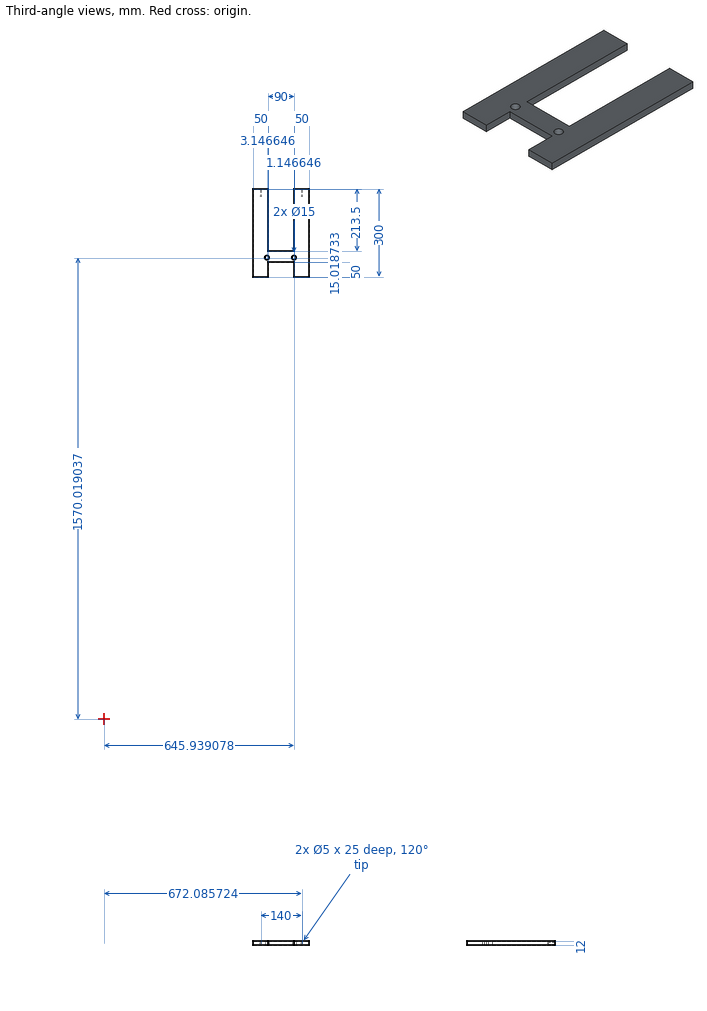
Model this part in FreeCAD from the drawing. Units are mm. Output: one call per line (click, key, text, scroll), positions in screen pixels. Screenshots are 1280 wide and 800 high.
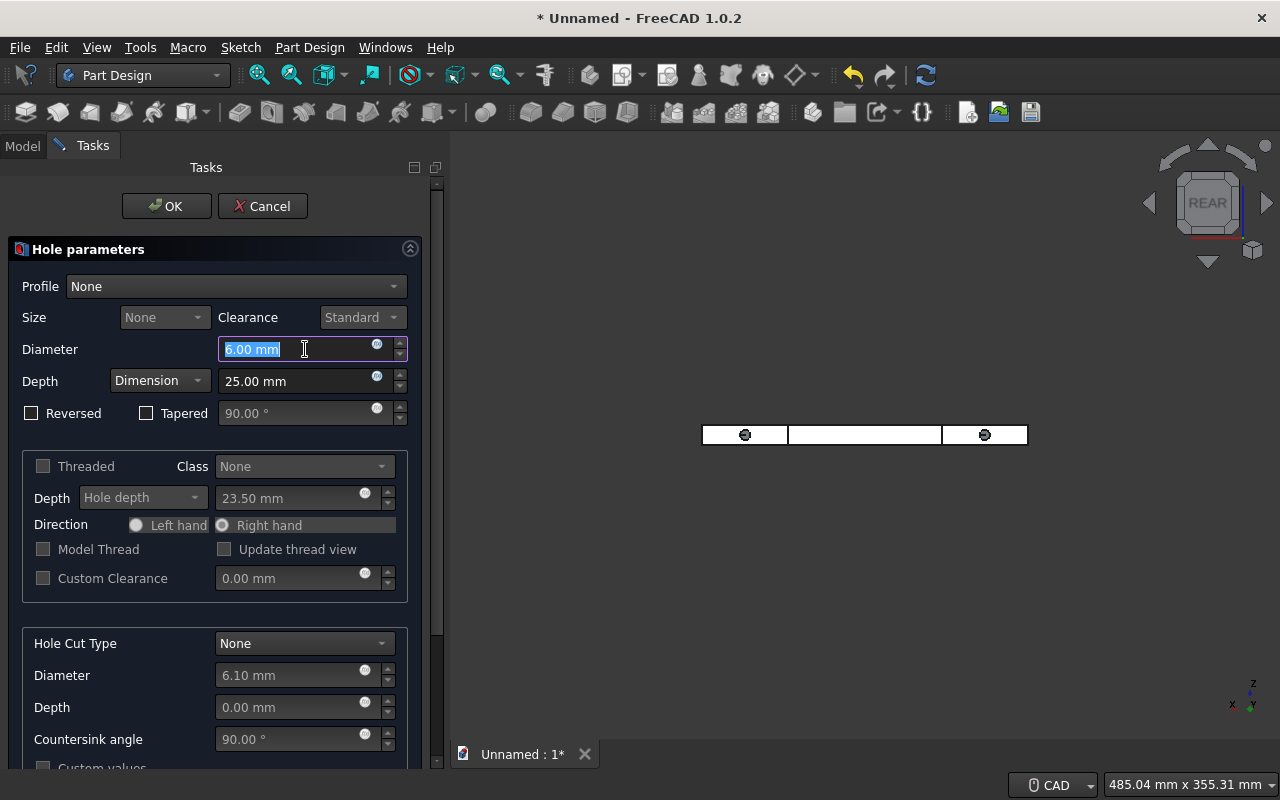
text(5)
key(Tab)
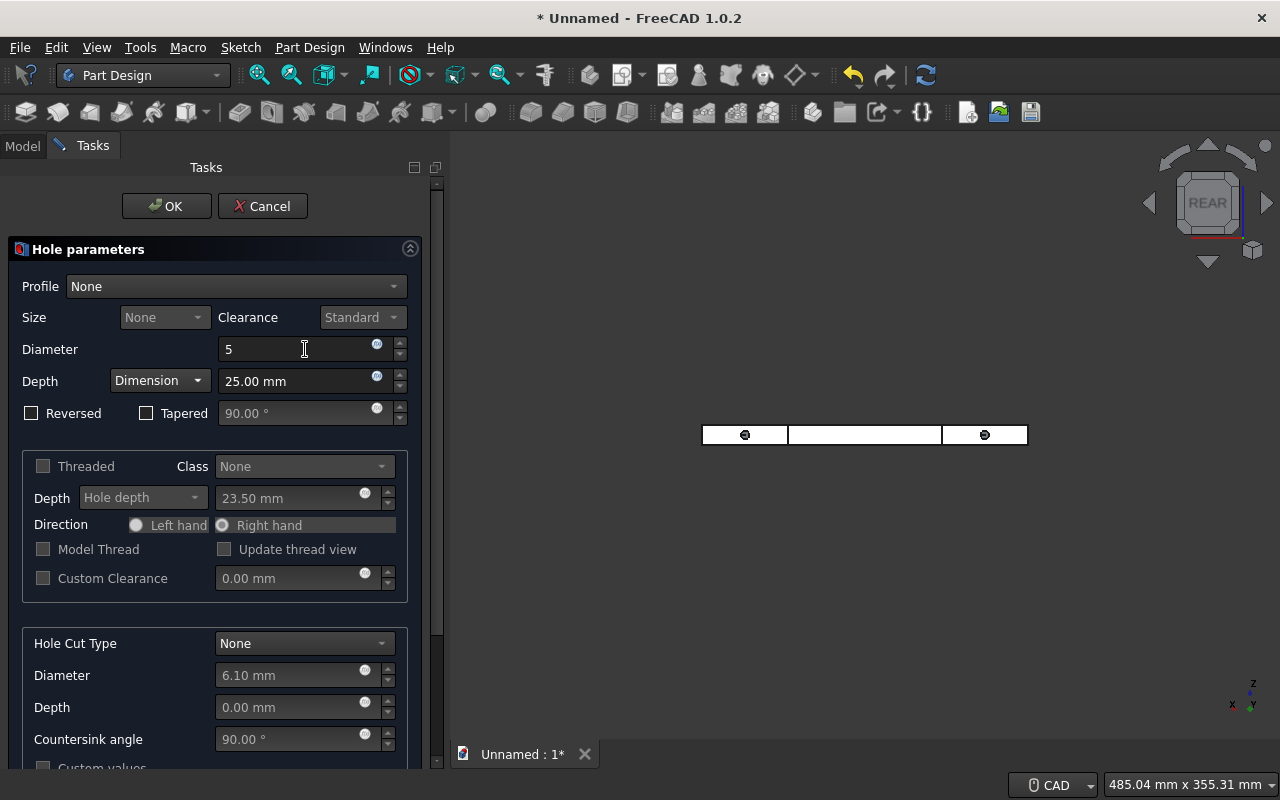
triple_click(305, 381)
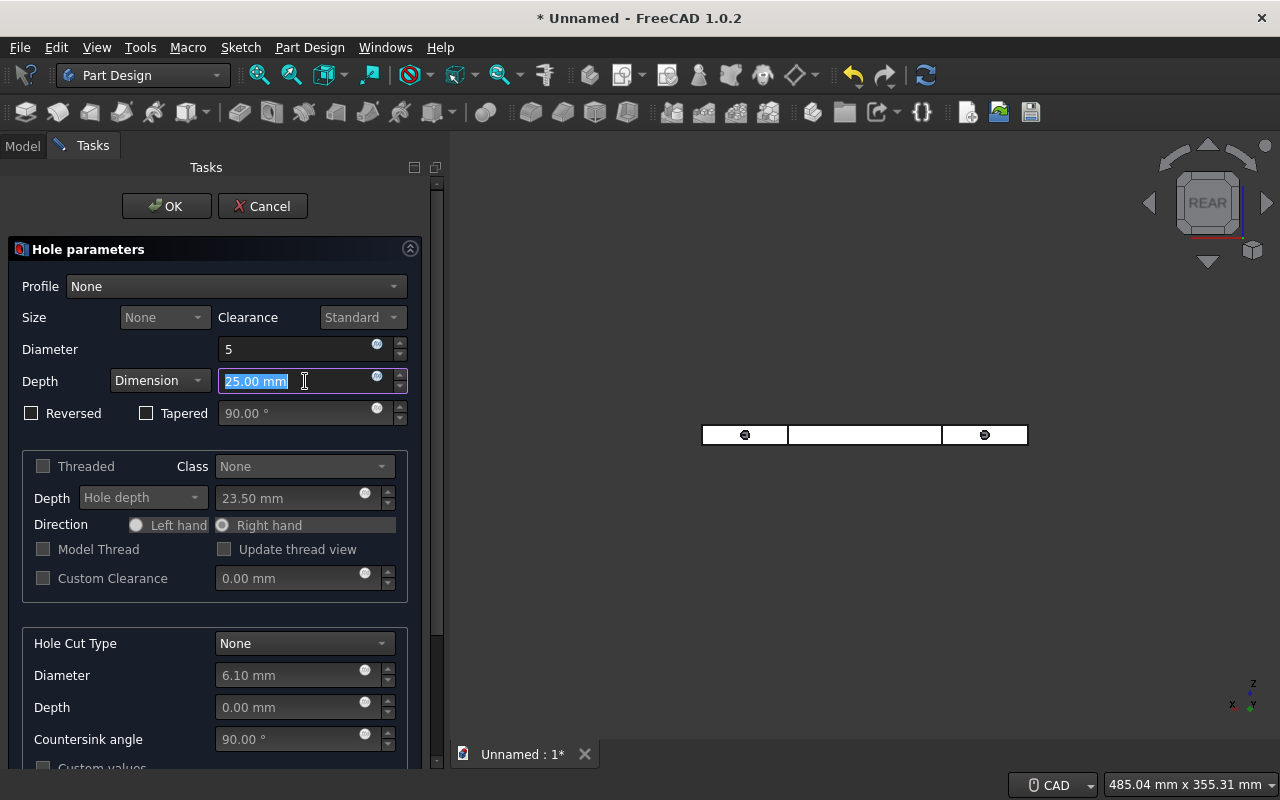
text(25)
key(Tab)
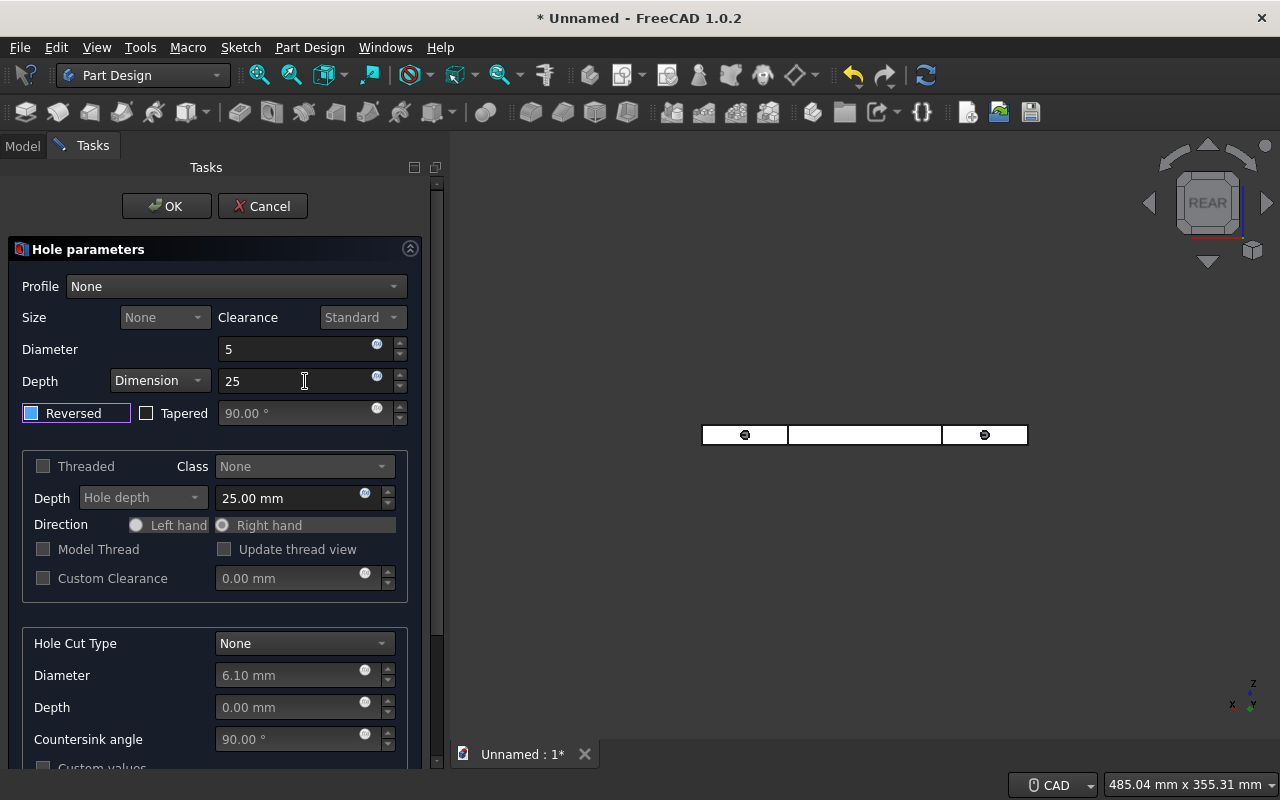
scroll(437, 472, down, 3)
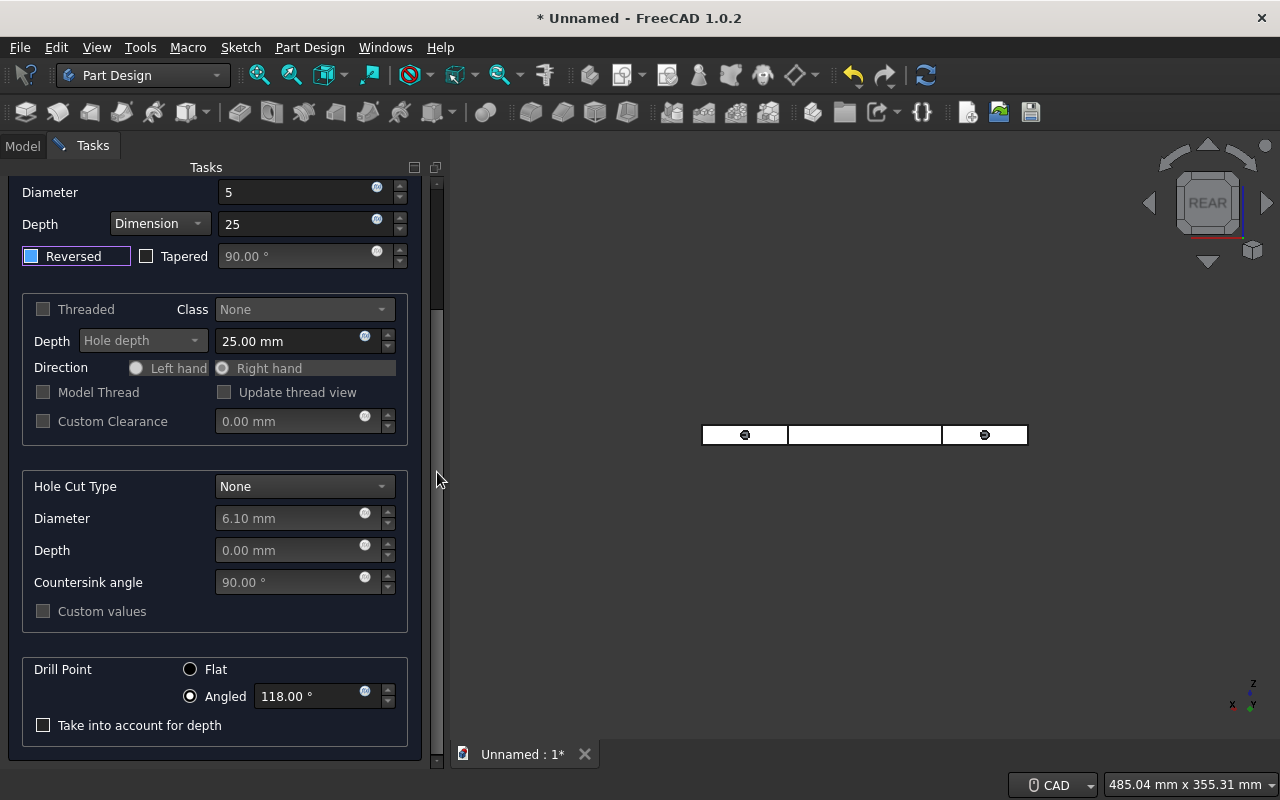
triple_click(317, 696)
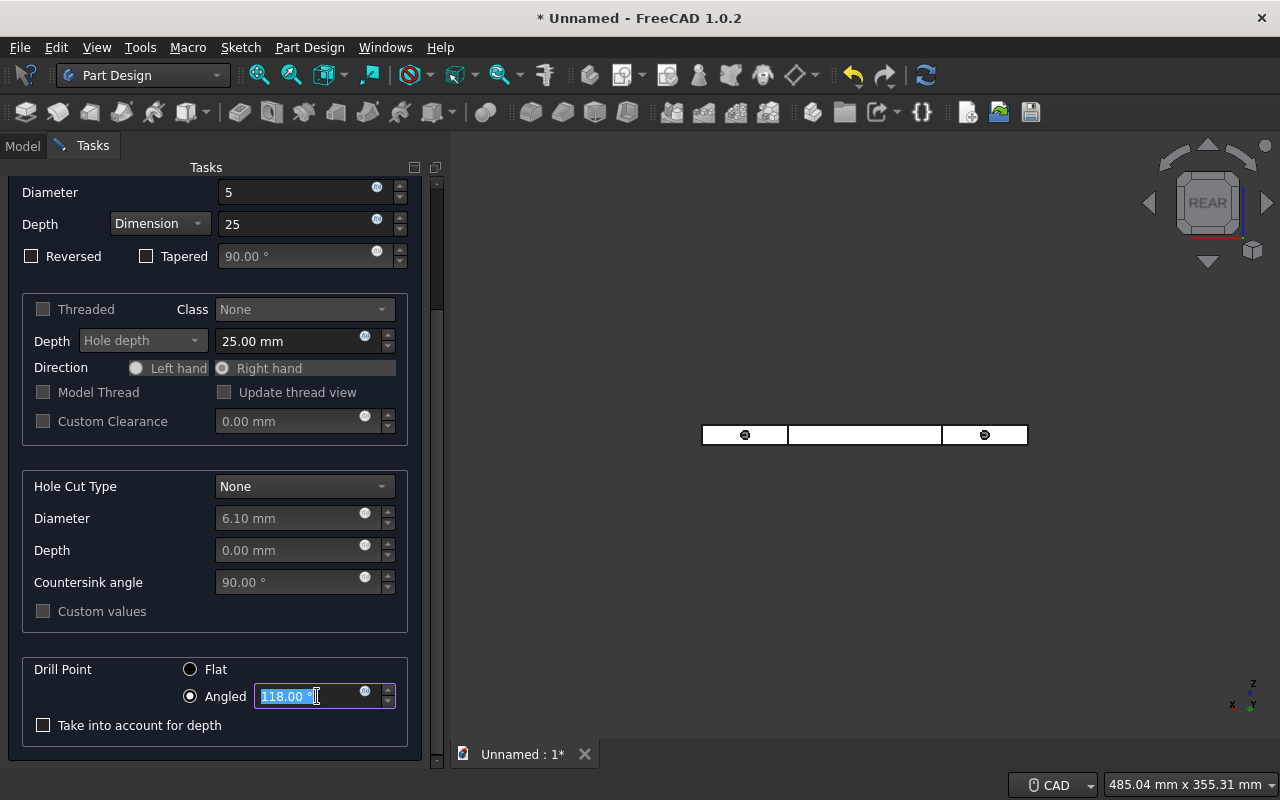
text(120)
key(Tab)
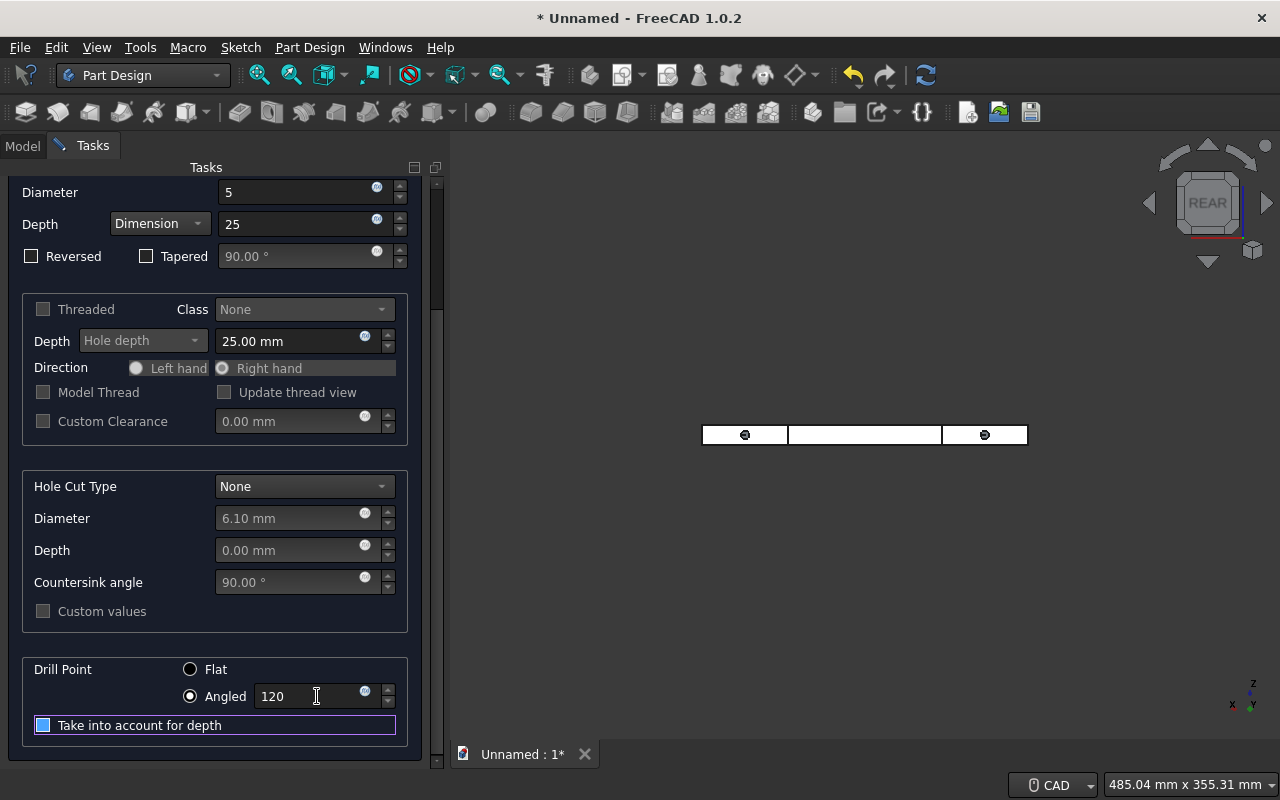
scroll(437, 472, up, 4)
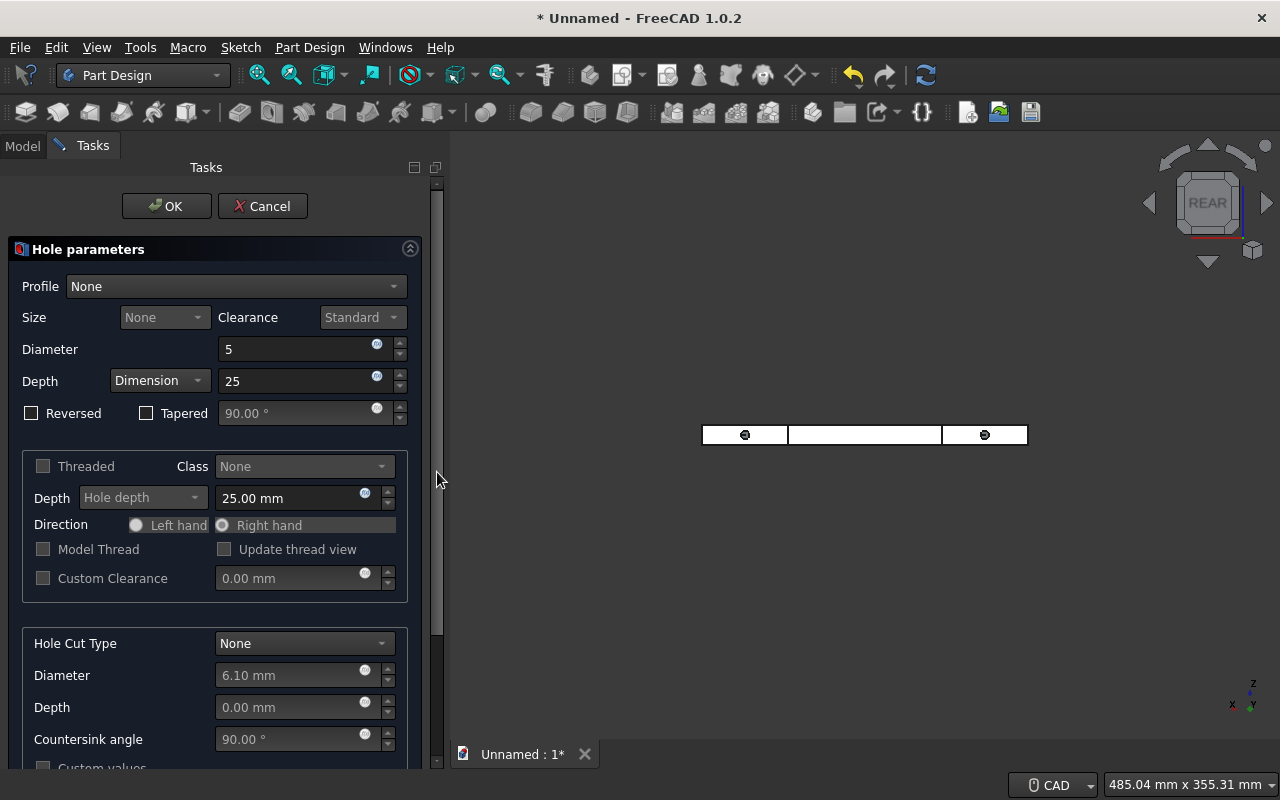
click(167, 206)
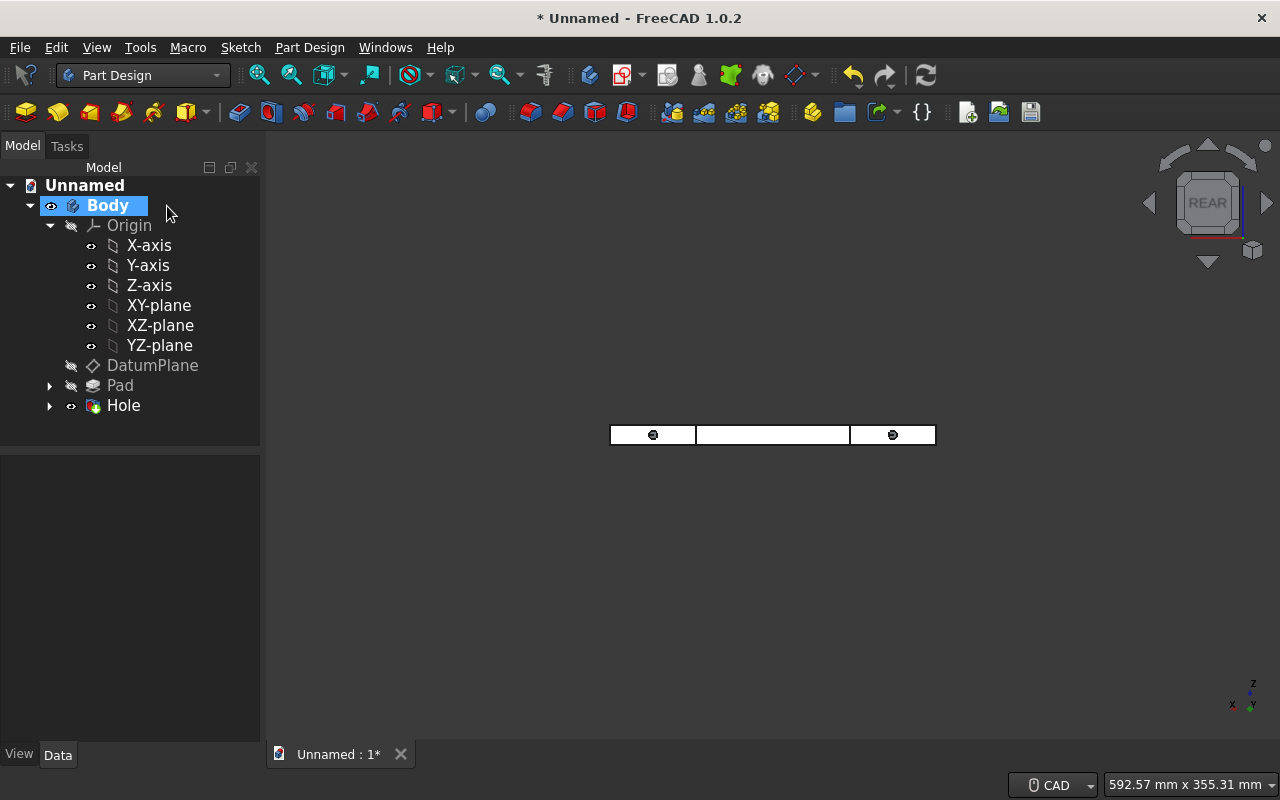
key(0)